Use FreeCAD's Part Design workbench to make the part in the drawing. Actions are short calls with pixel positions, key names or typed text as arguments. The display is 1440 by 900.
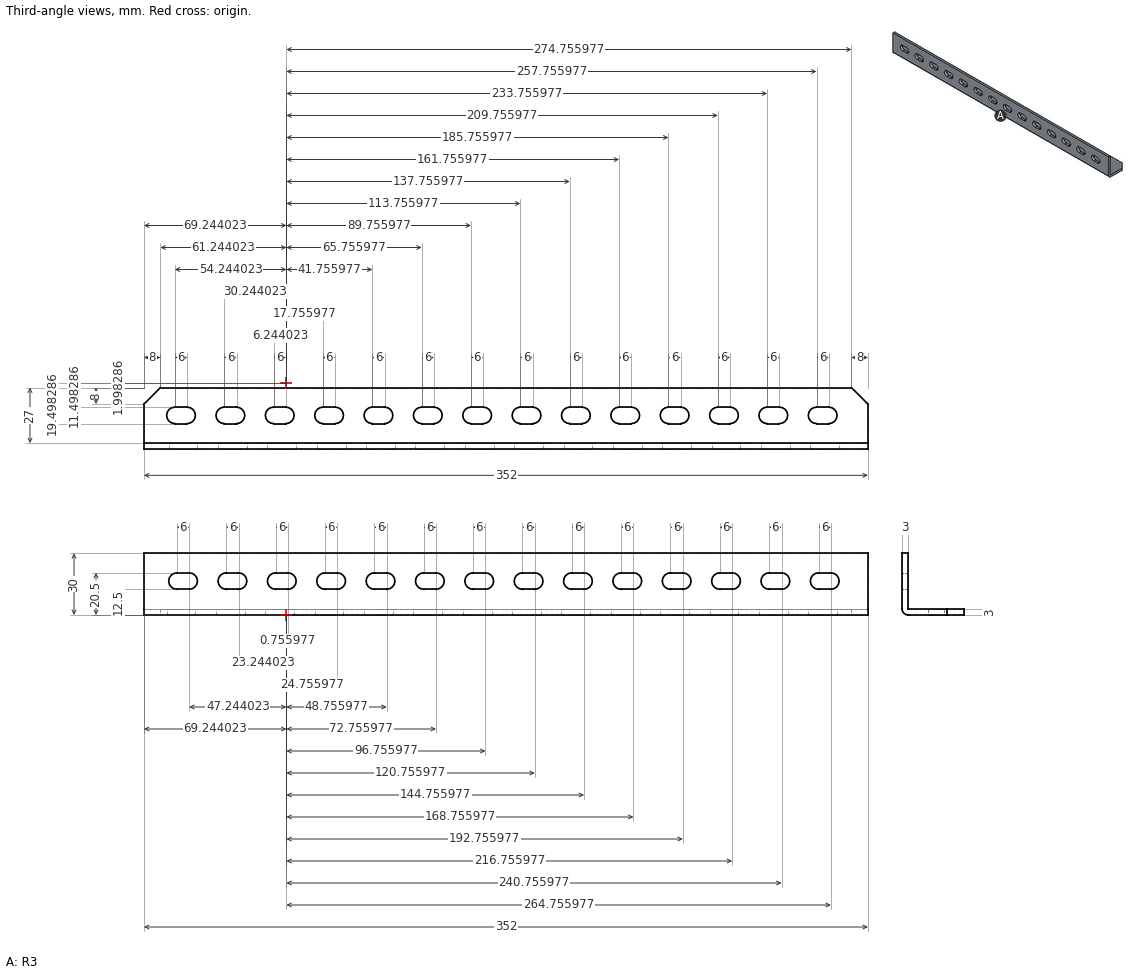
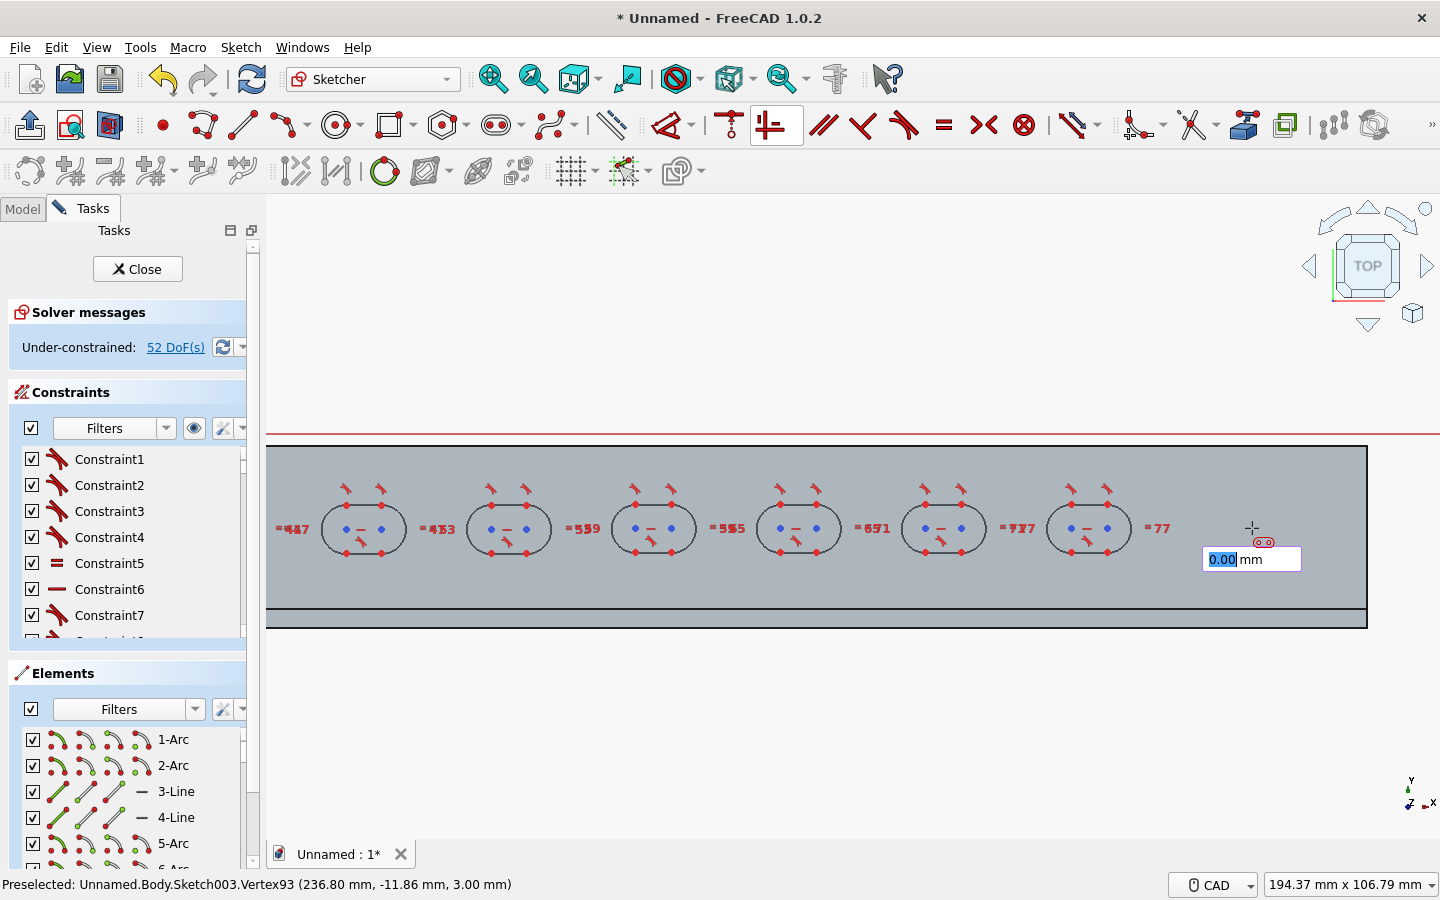
click(1234, 504)
key(Escape)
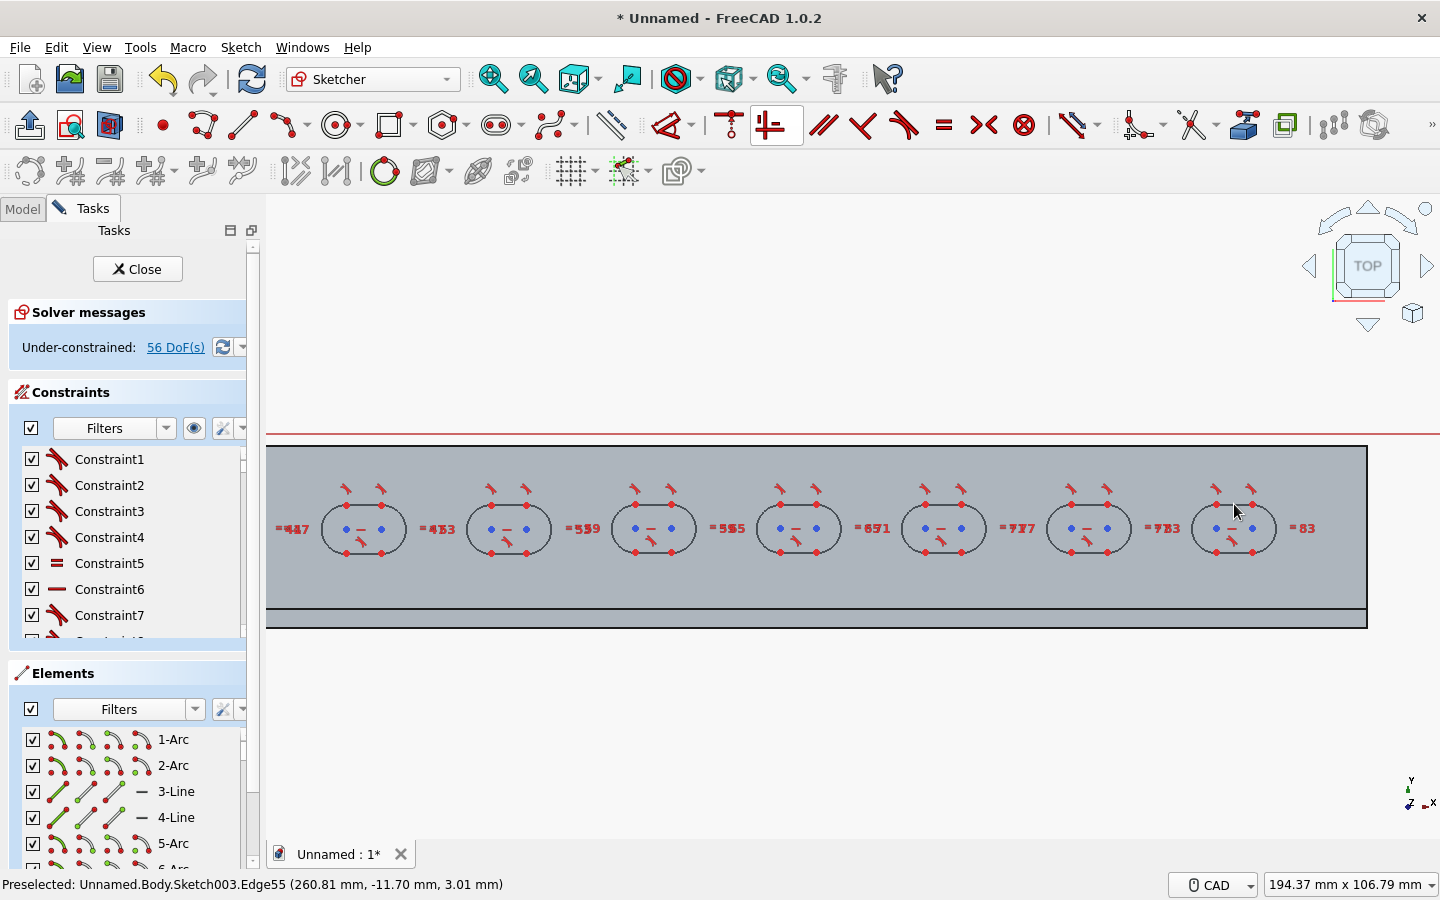
scroll(1071, 530, down, 5)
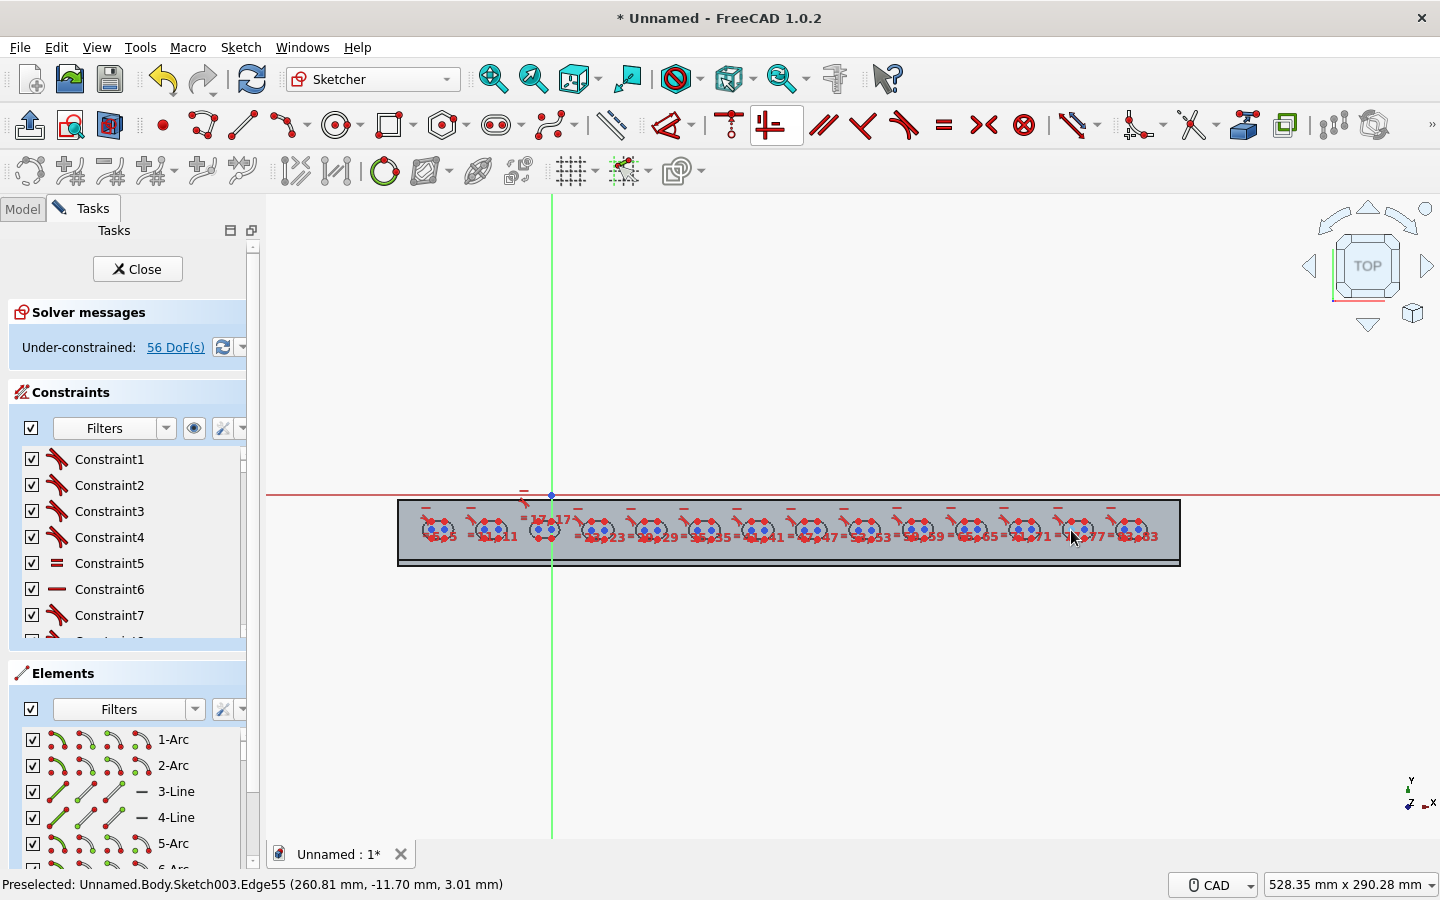
scroll(424, 525, up, 3)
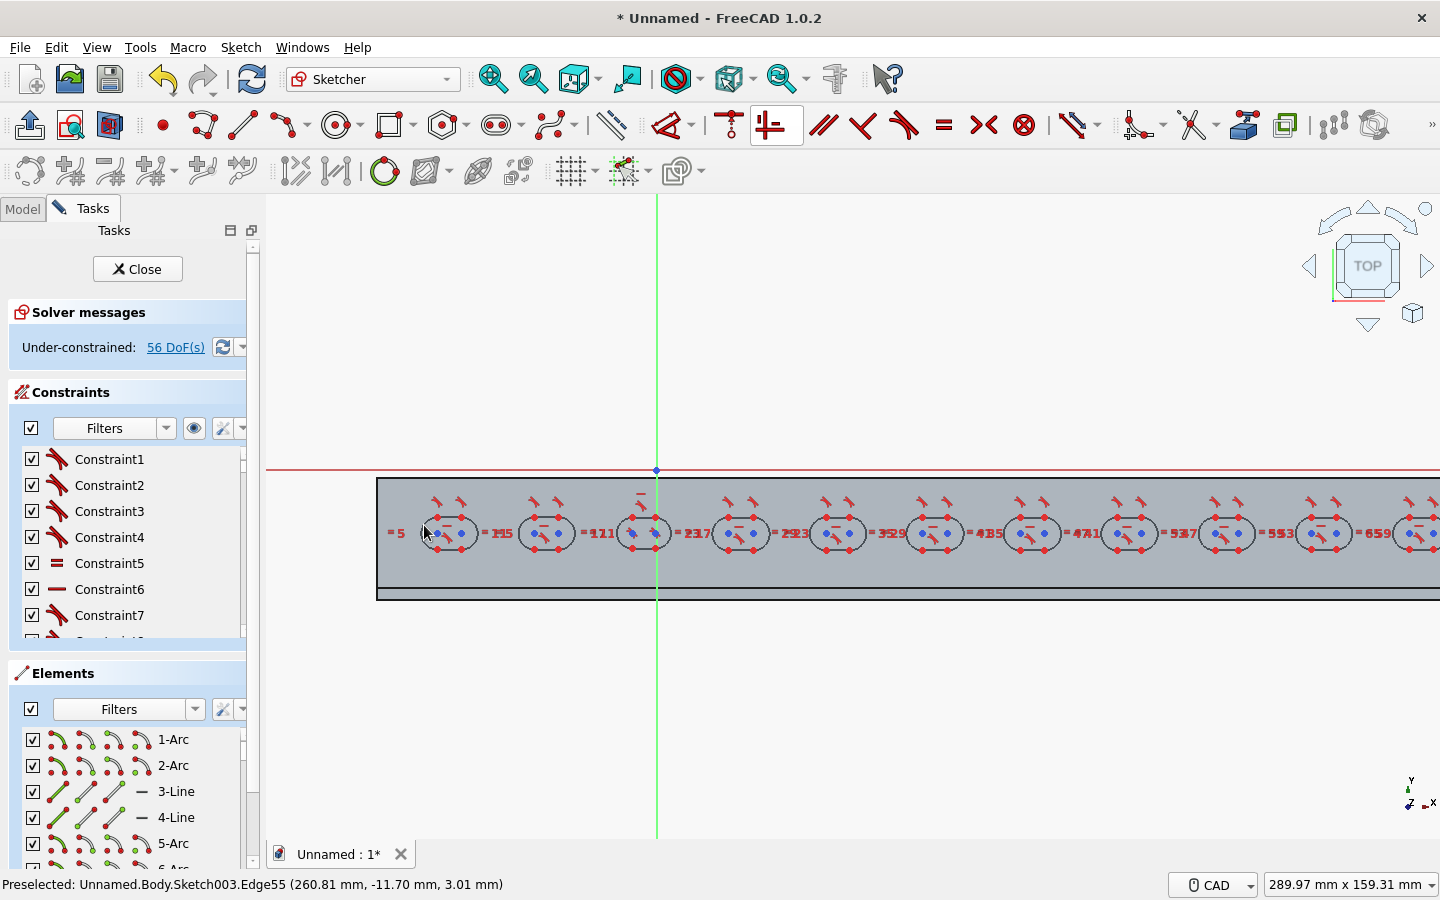
click(424, 524)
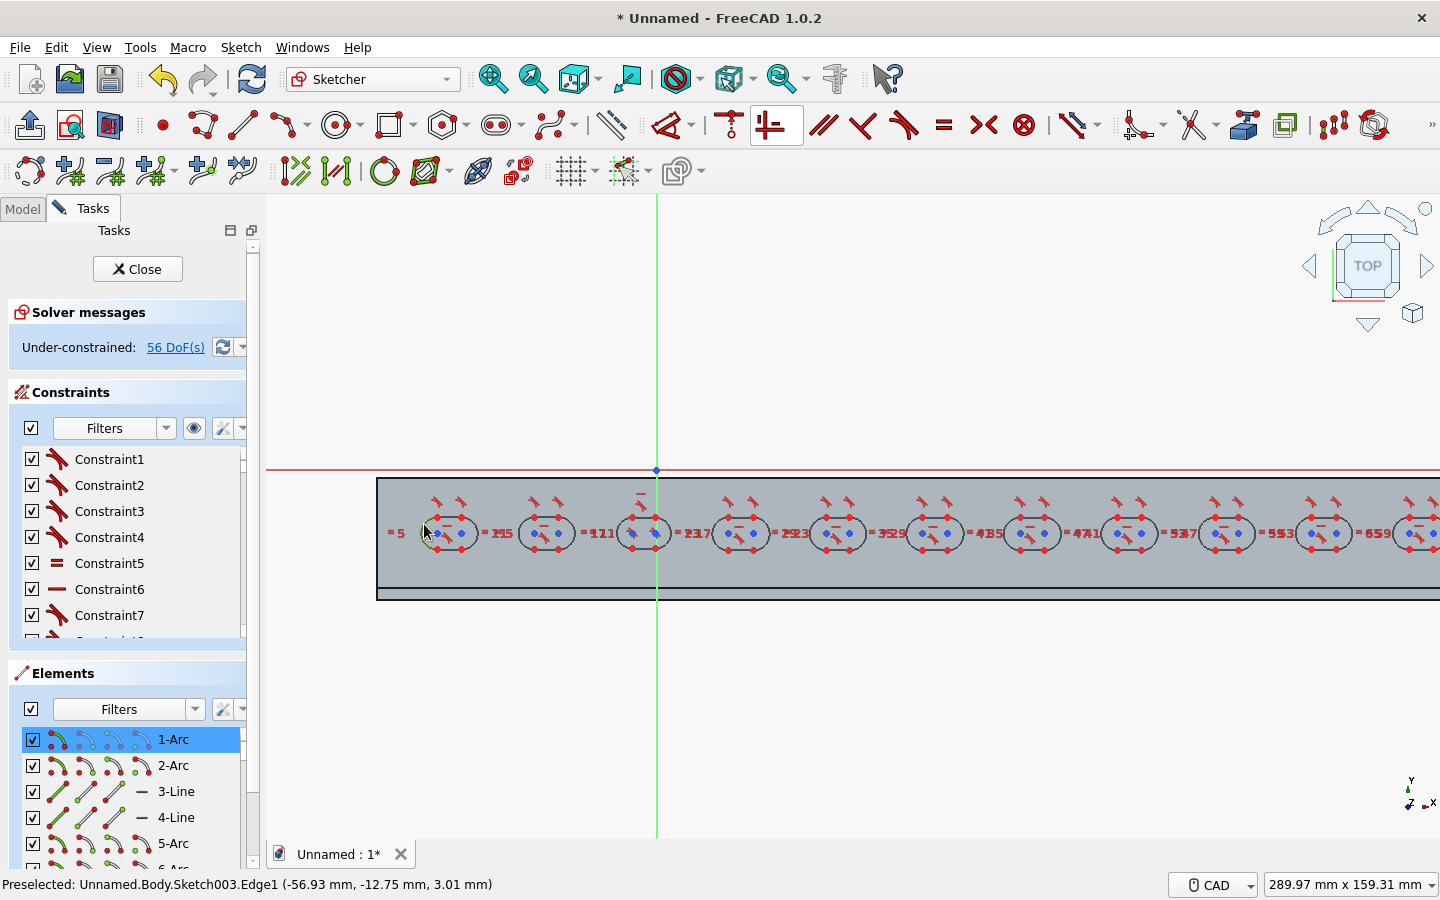
click(522, 524)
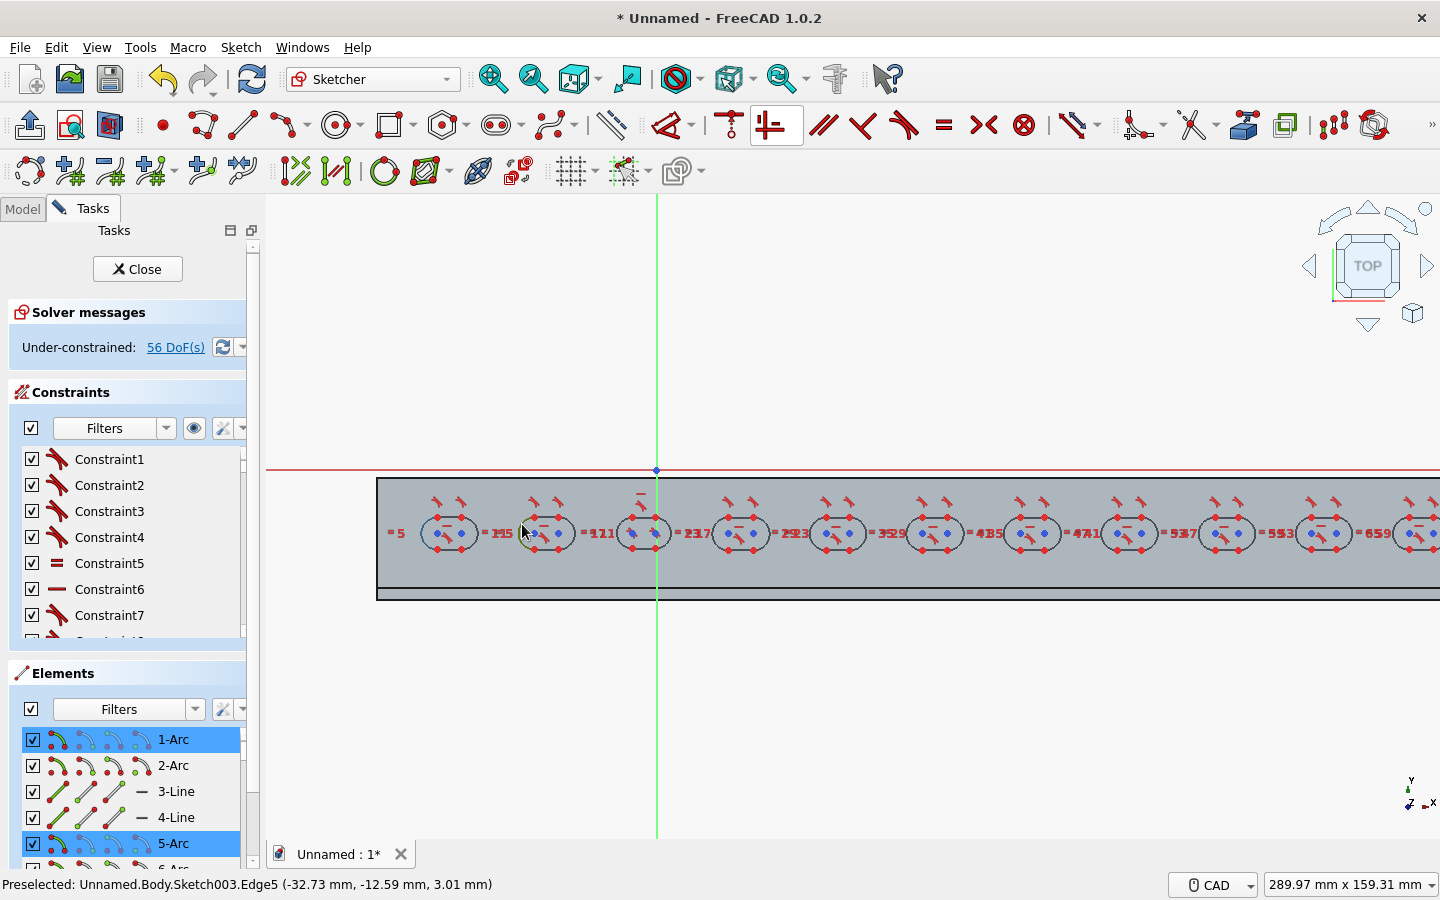
click(620, 524)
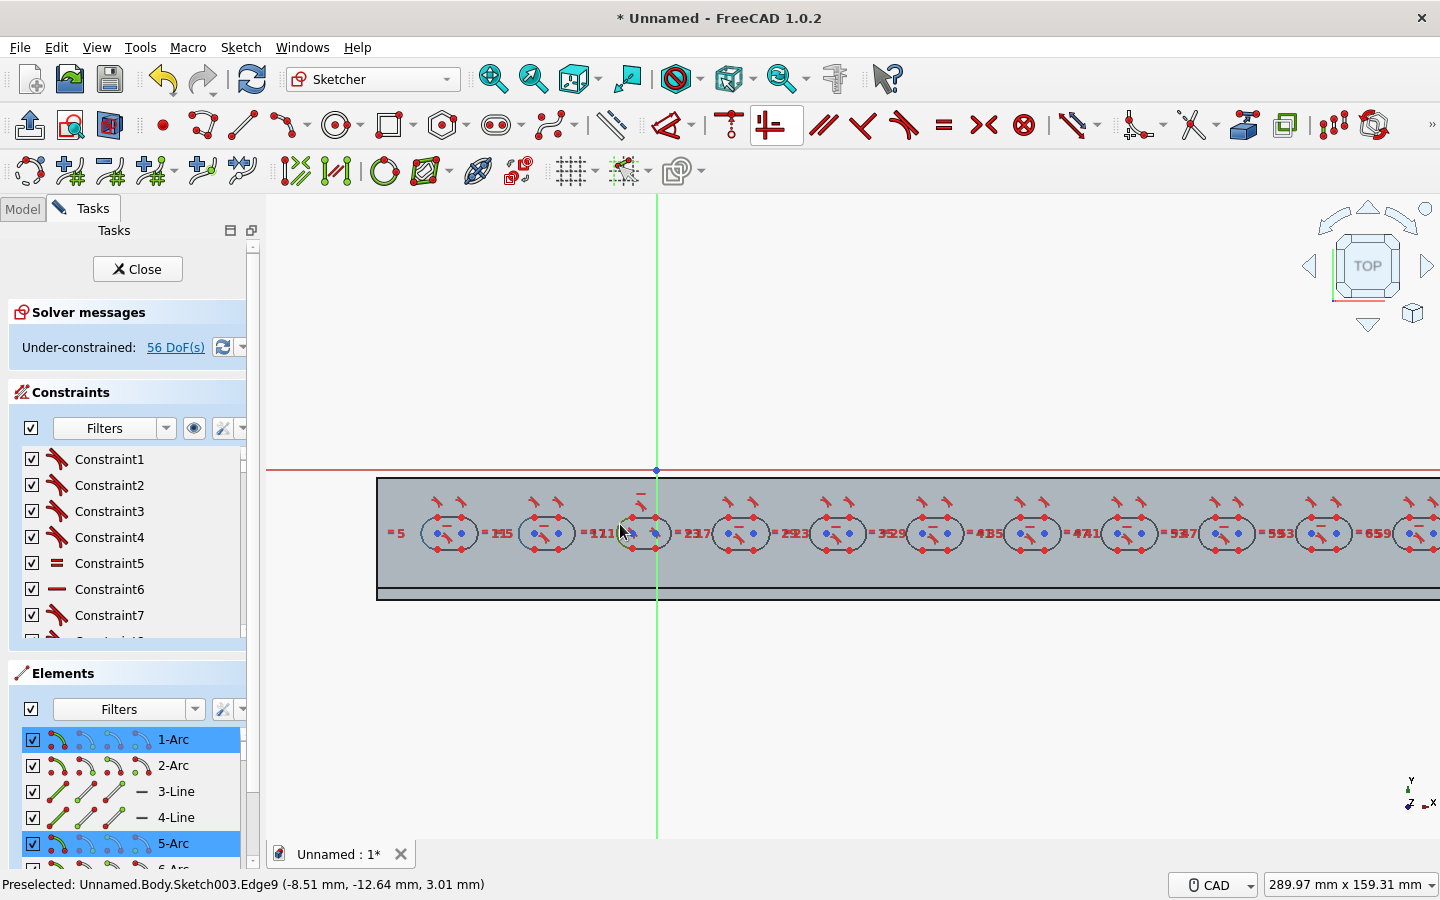
click(715, 524)